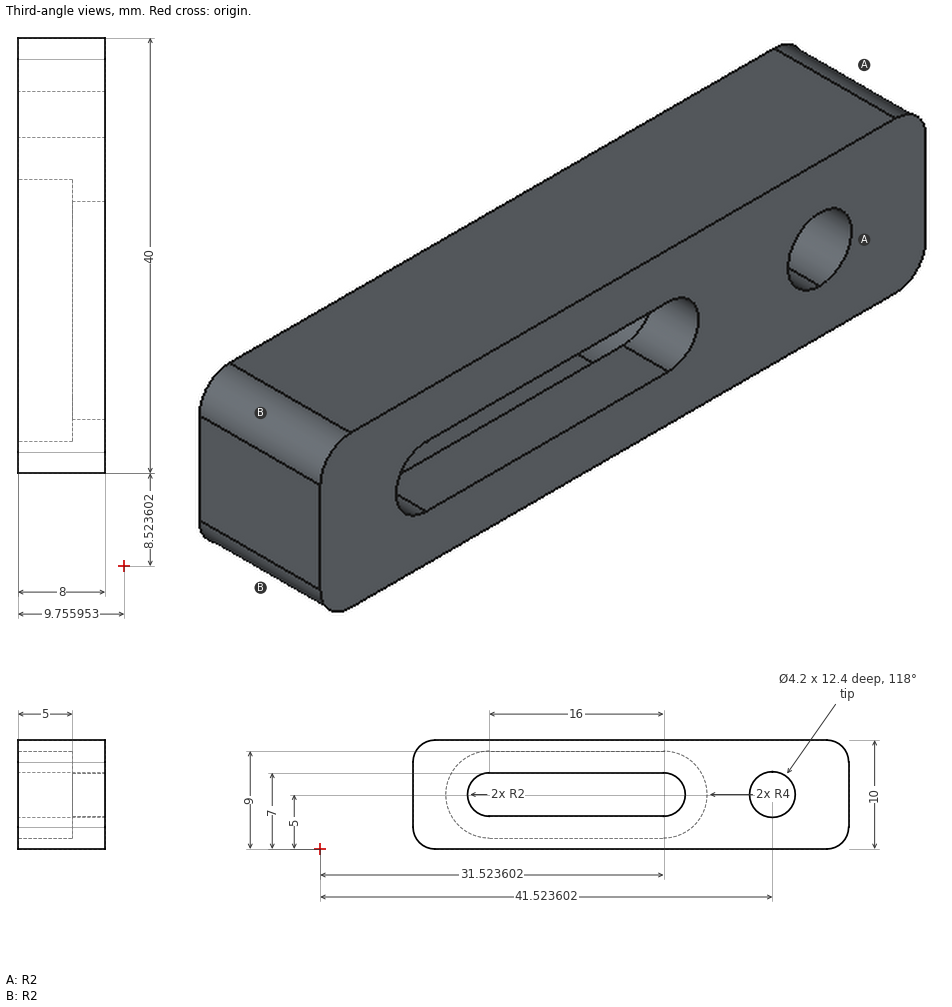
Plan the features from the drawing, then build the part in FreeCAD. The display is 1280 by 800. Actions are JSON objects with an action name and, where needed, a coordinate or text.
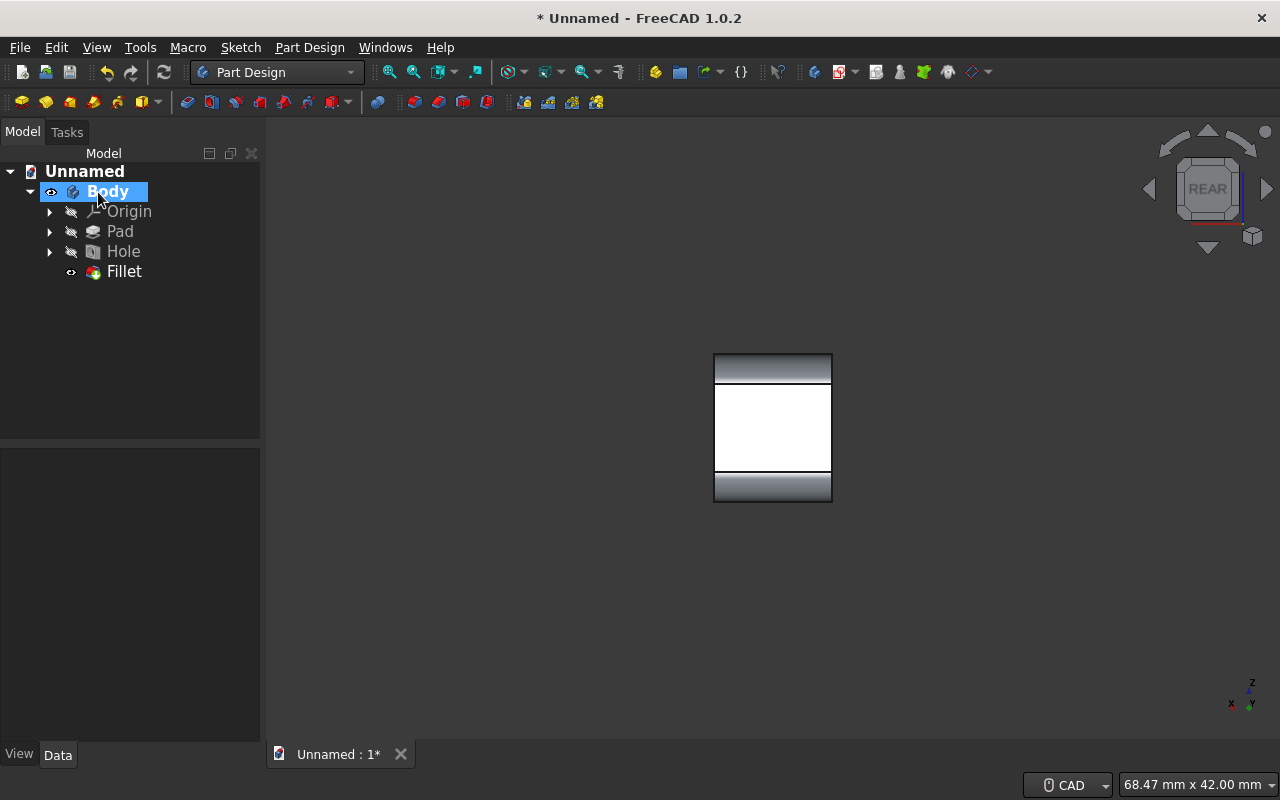
{"action": "left_click", "coordinate": [390, 72]}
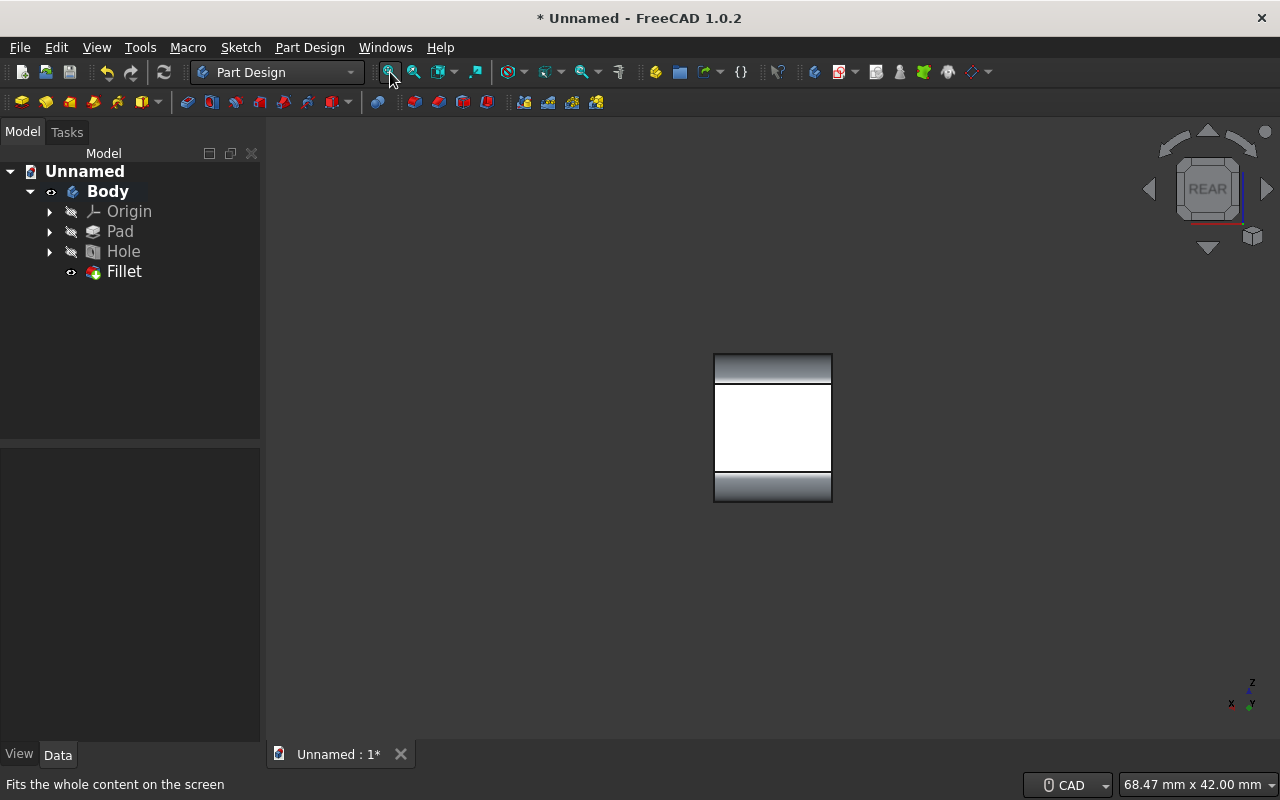
{"action": "key", "text": "6"}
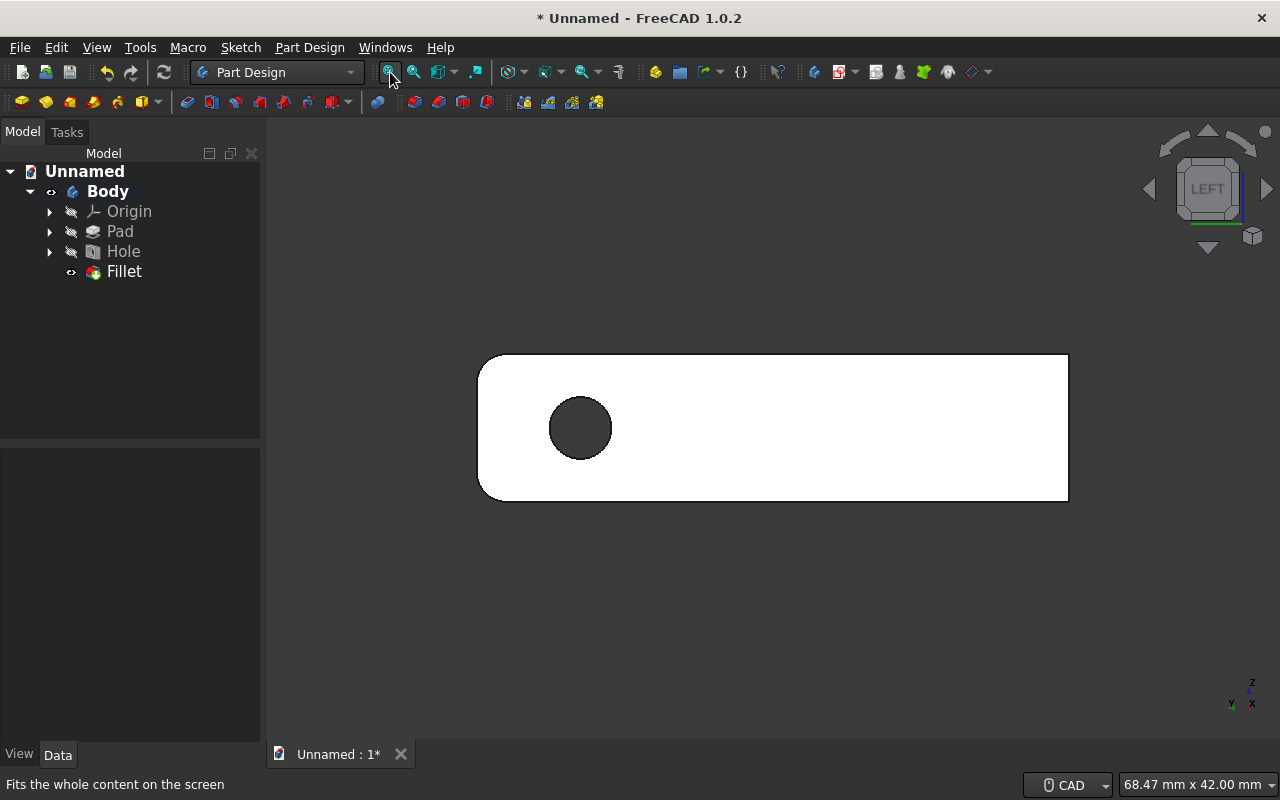
{"action": "left_click", "coordinate": [688, 427]}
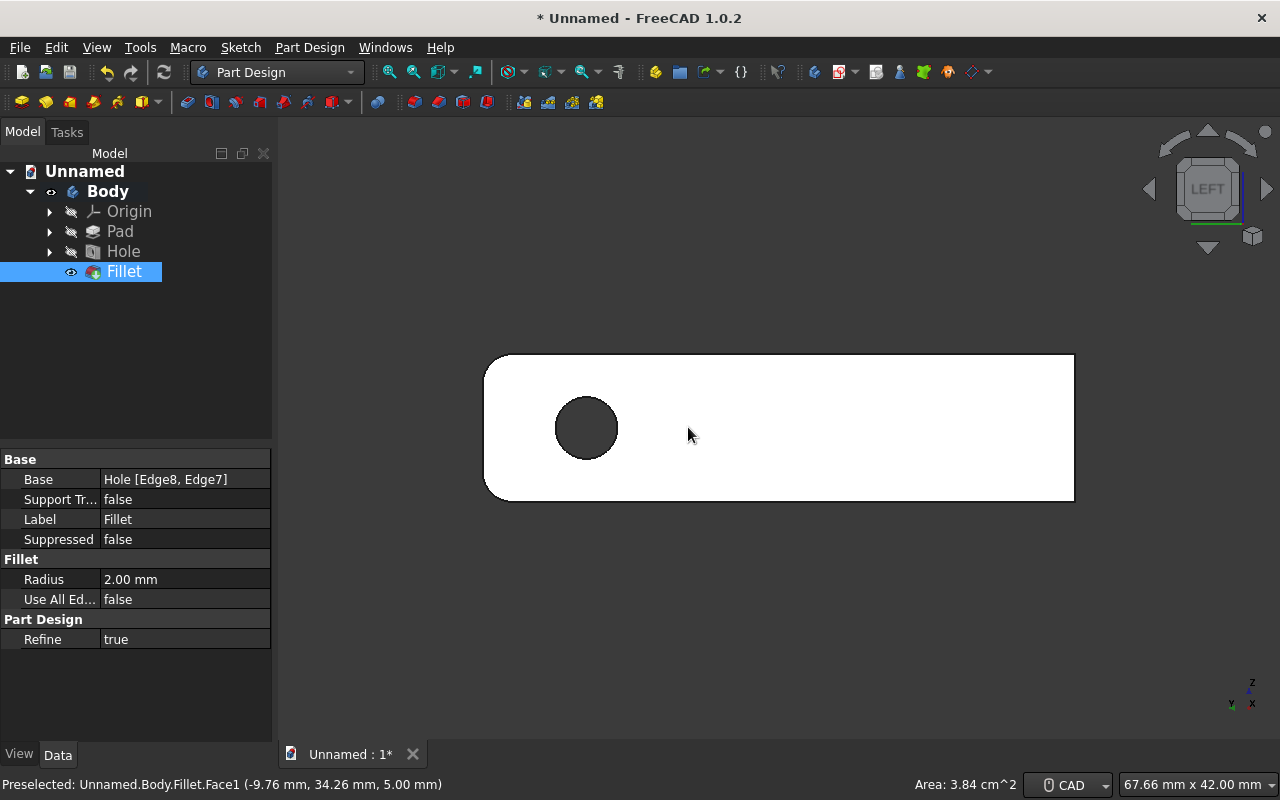
{"action": "left_click", "coordinate": [840, 72]}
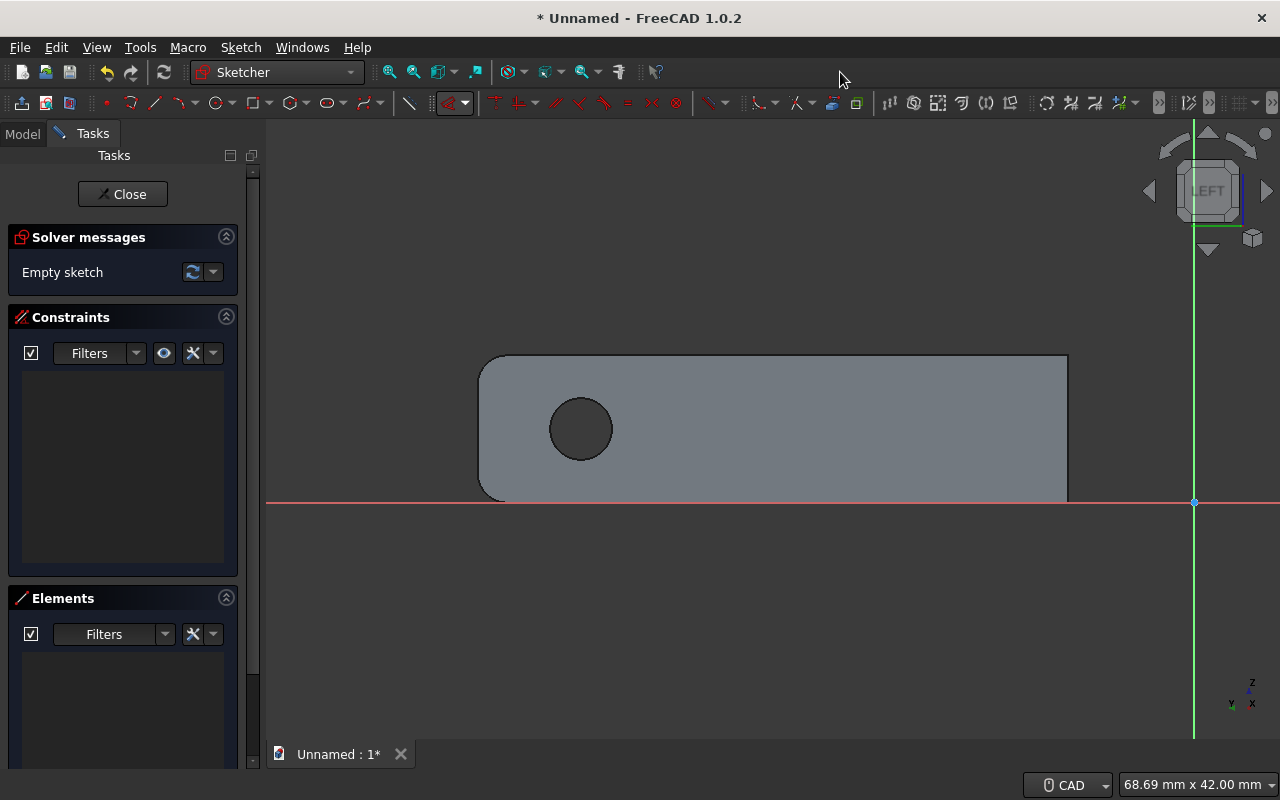
{"action": "scroll", "coordinate": [294, 329], "scroll_direction": "down", "scroll_amount": 1}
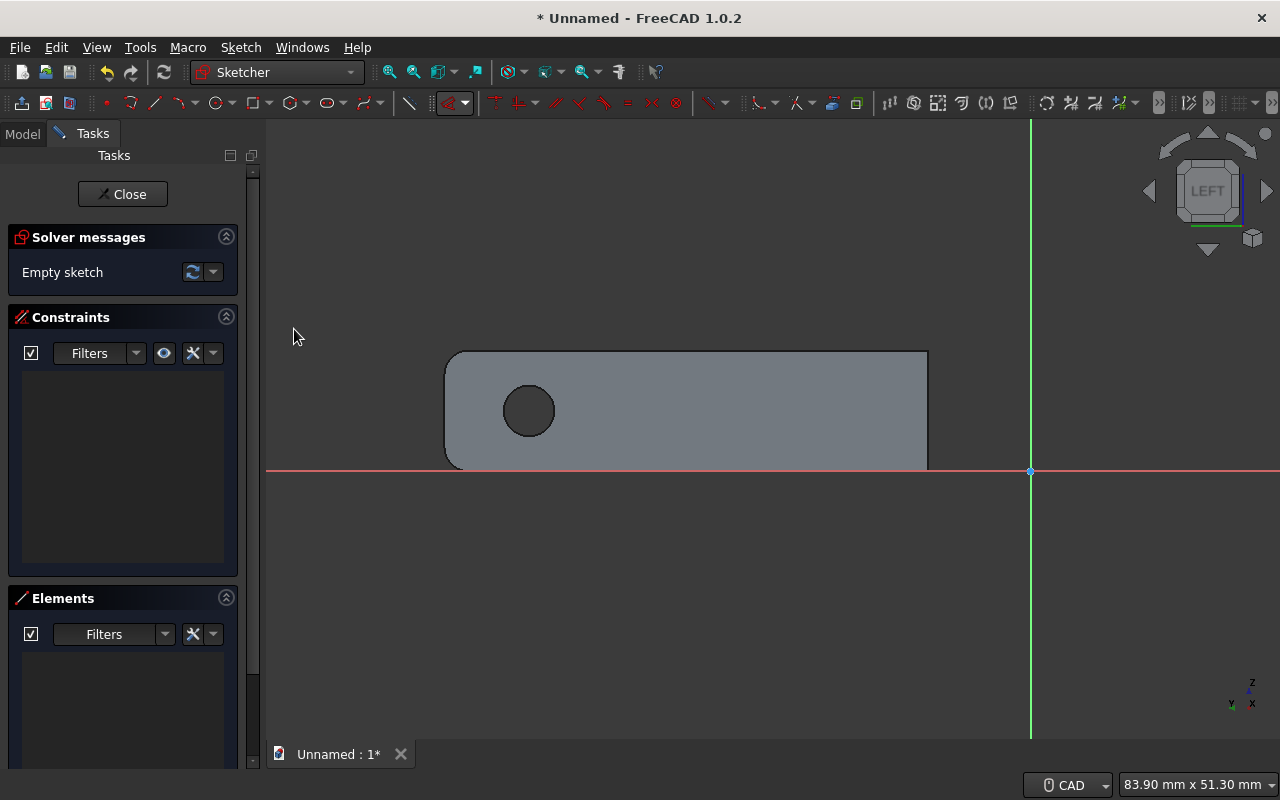
{"action": "scroll", "coordinate": [1080, 429], "scroll_direction": "up", "scroll_amount": 2}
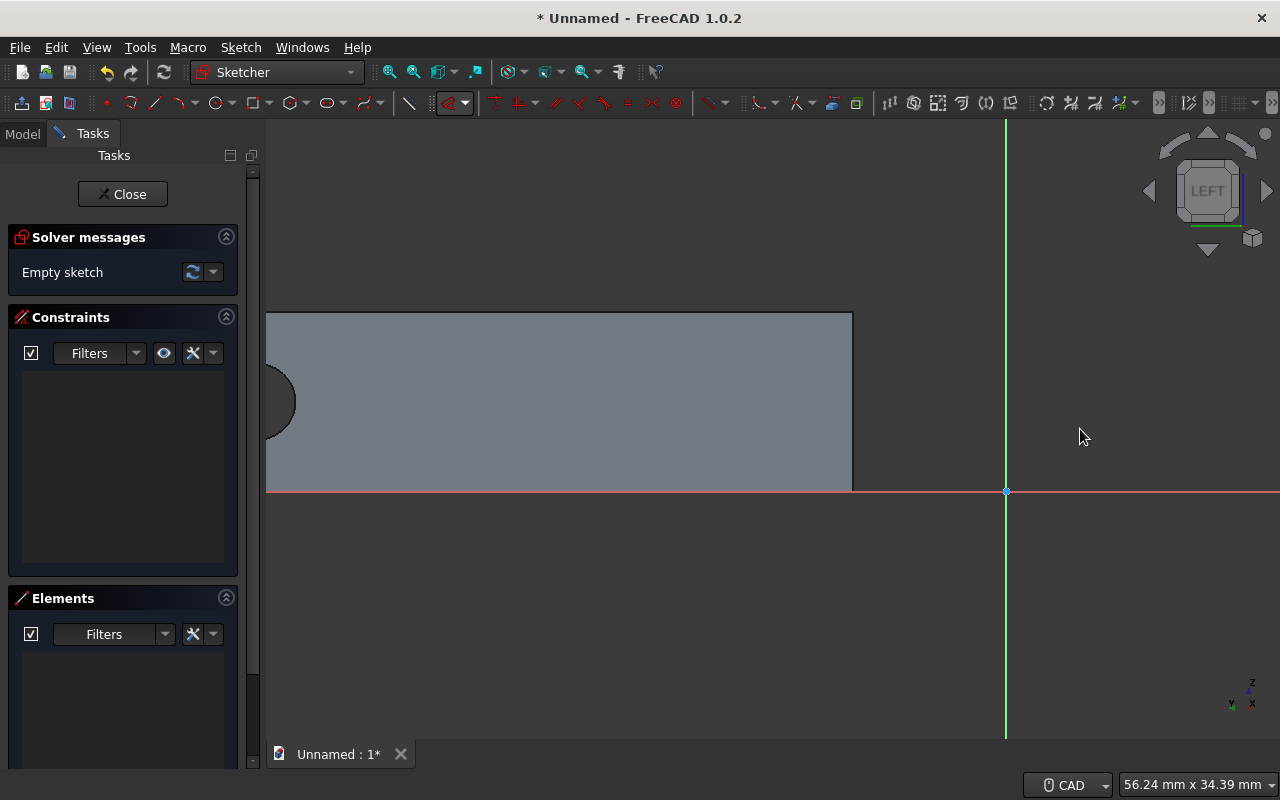
{"action": "key", "text": "g s"}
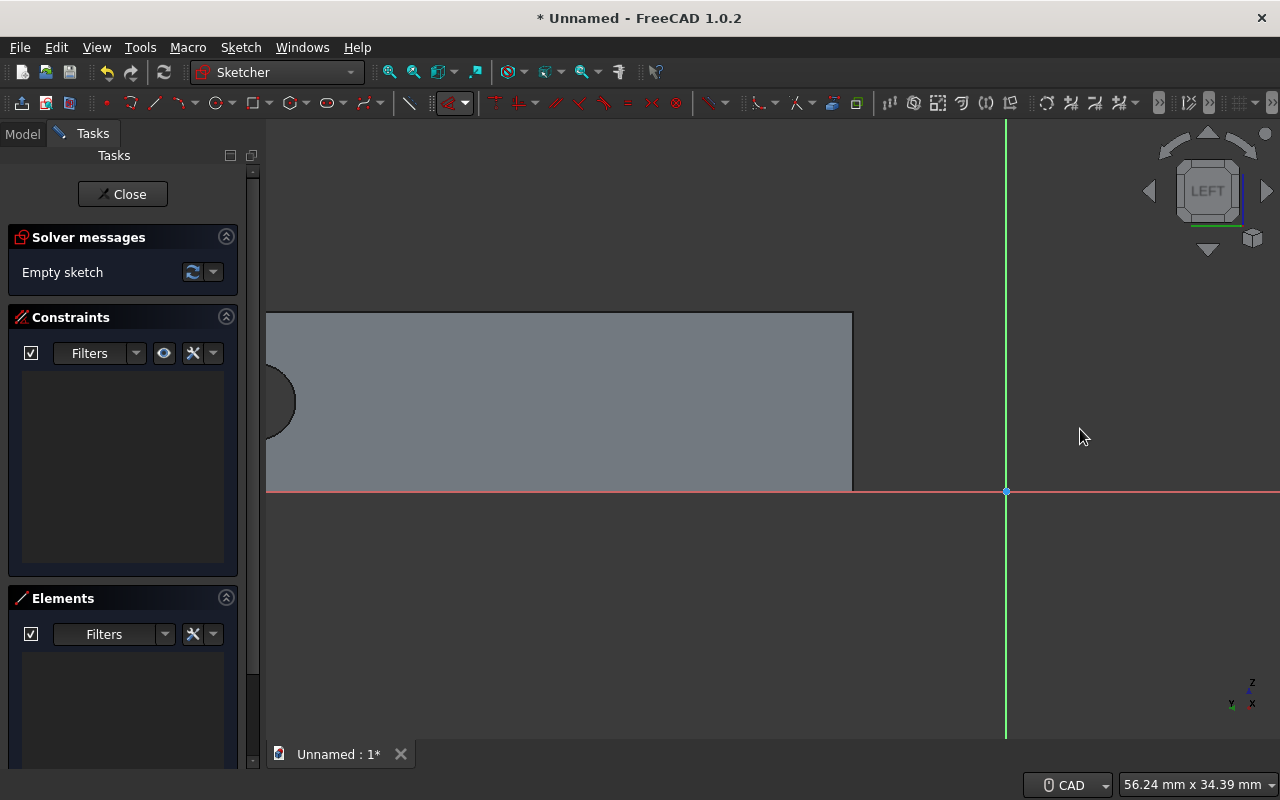
{"action": "left_click", "coordinate": [438, 402]}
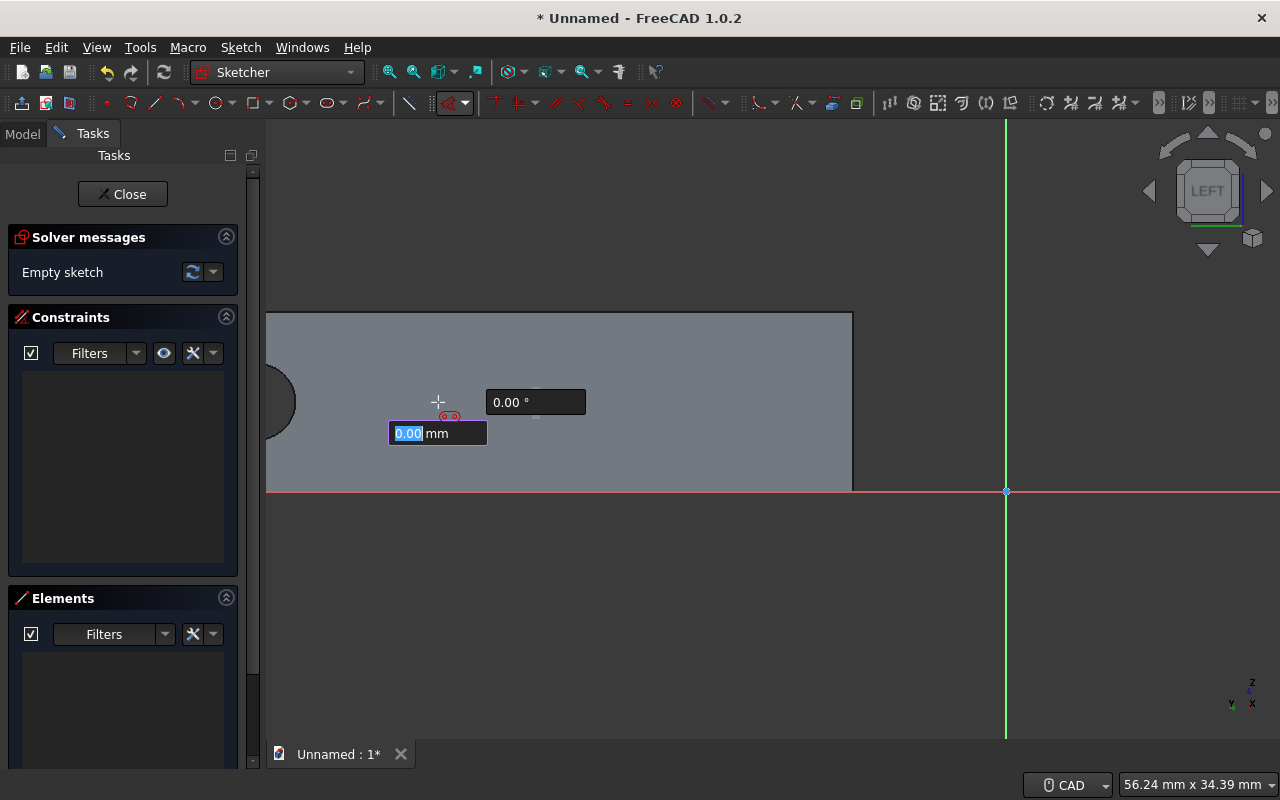
{"action": "left_click", "coordinate": [726, 402]}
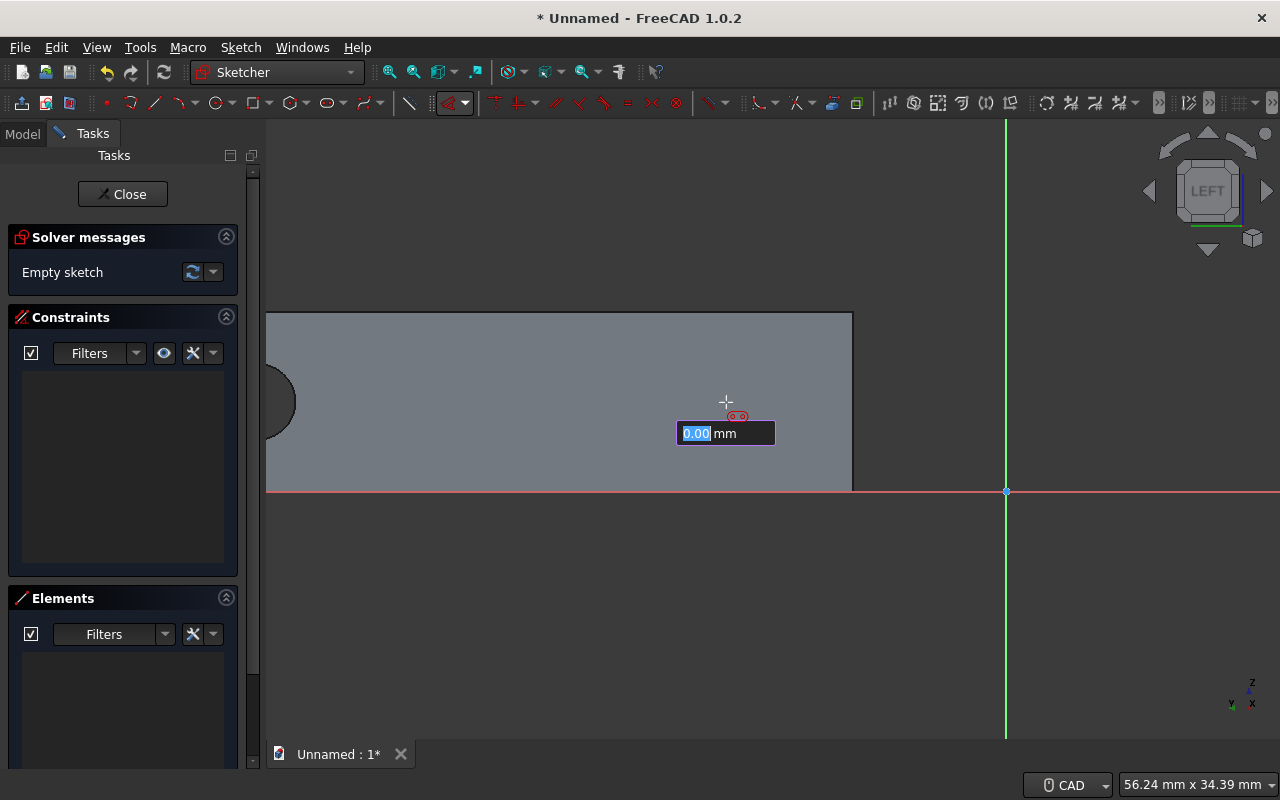
{"action": "left_click", "coordinate": [582, 438]}
{"action": "key", "text": "Escape"}